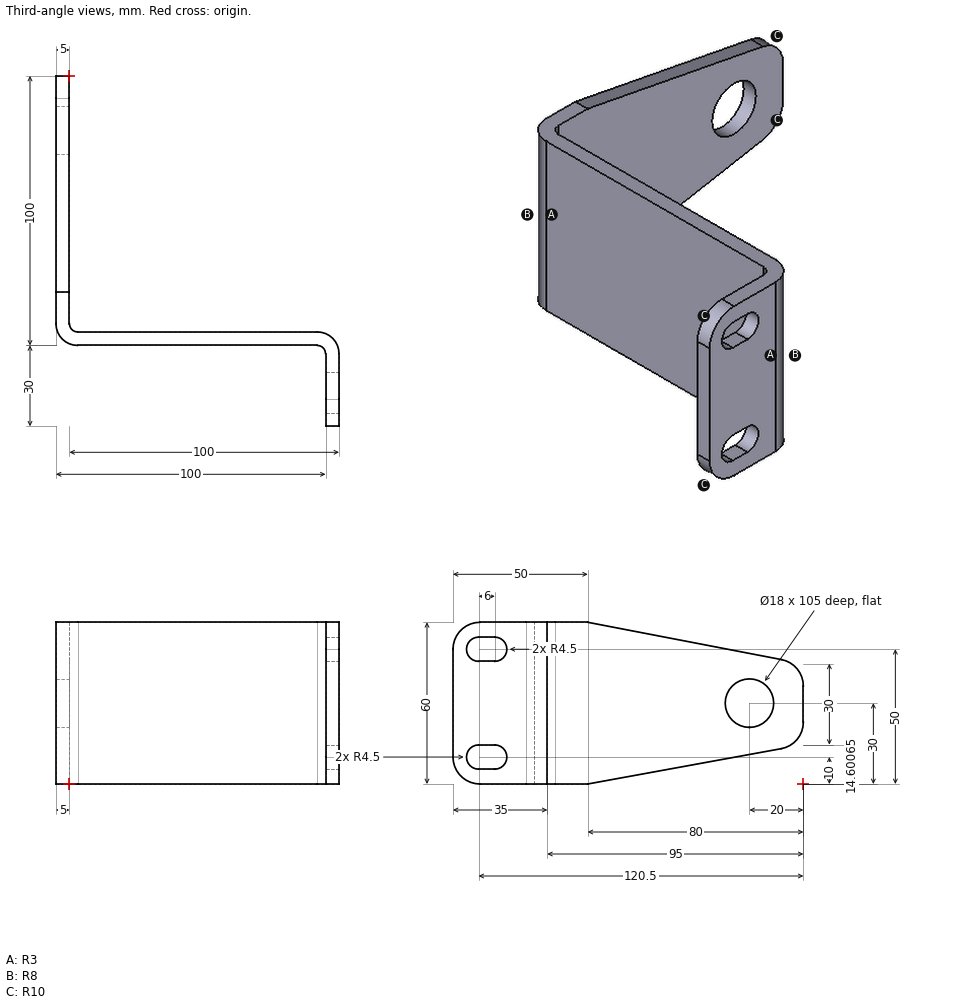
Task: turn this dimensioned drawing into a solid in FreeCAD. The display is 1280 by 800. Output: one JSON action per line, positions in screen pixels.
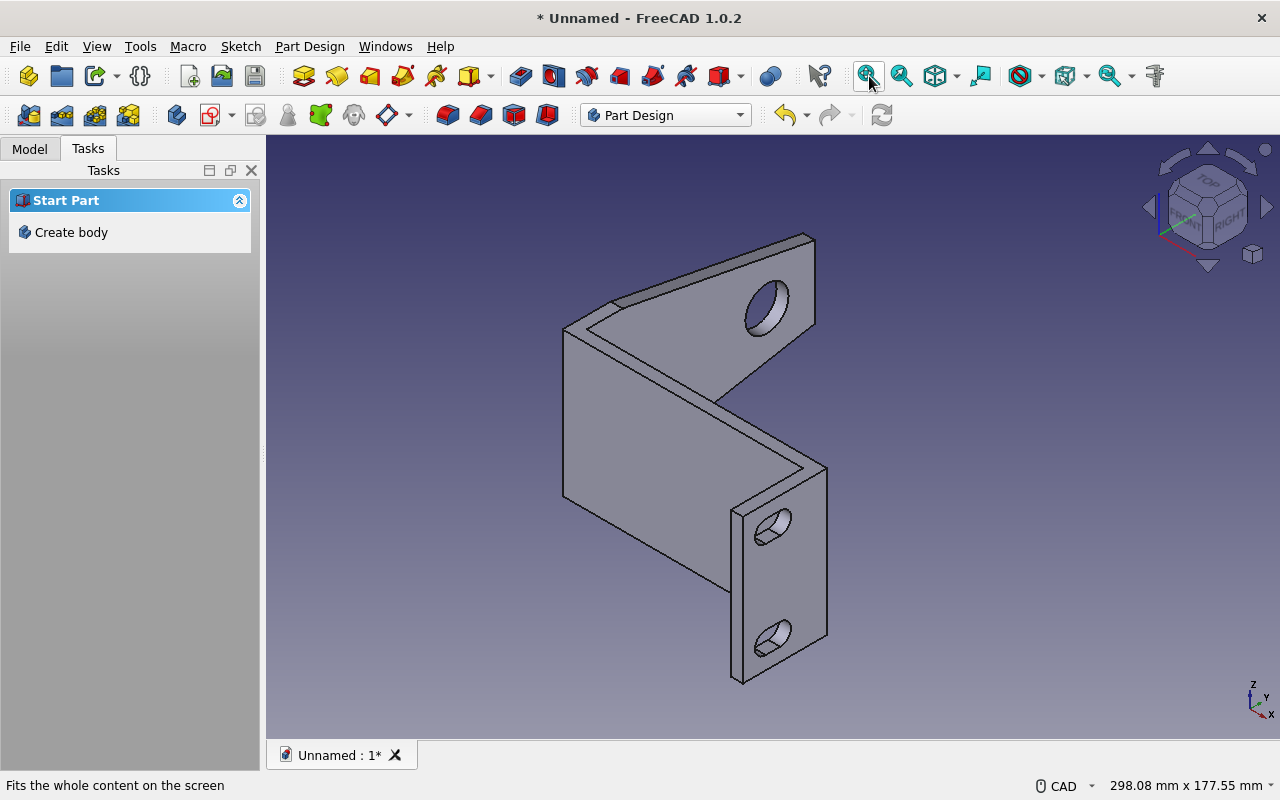
{"action": "key", "text": "2"}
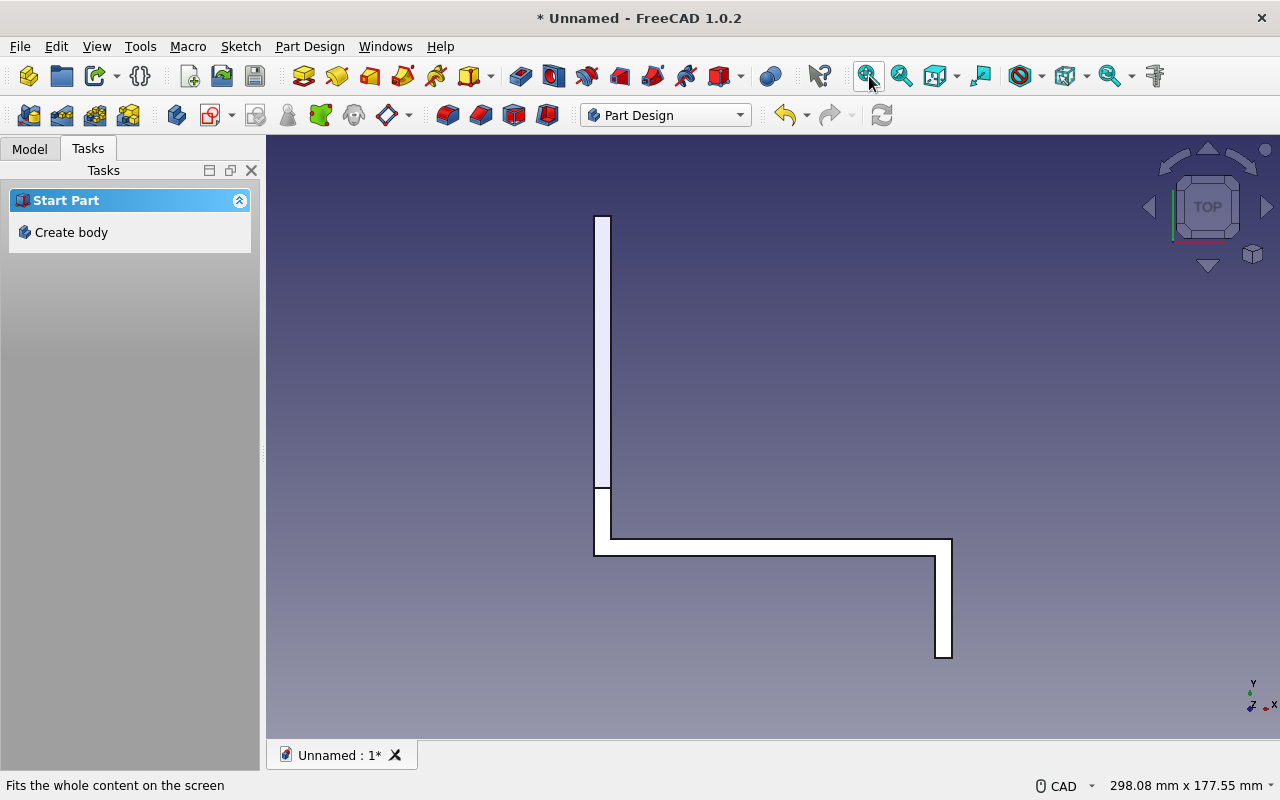
{"action": "key", "text": "1"}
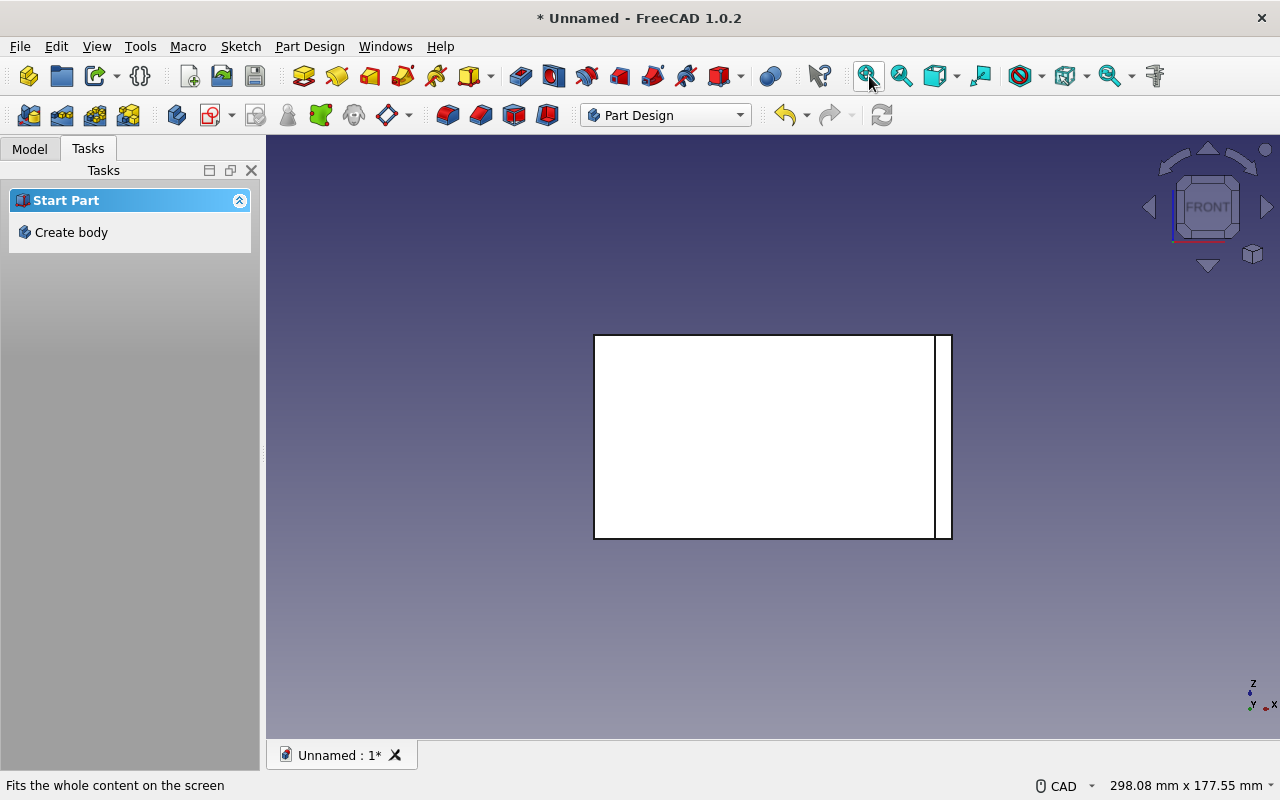
{"action": "left_click", "coordinate": [869, 76]}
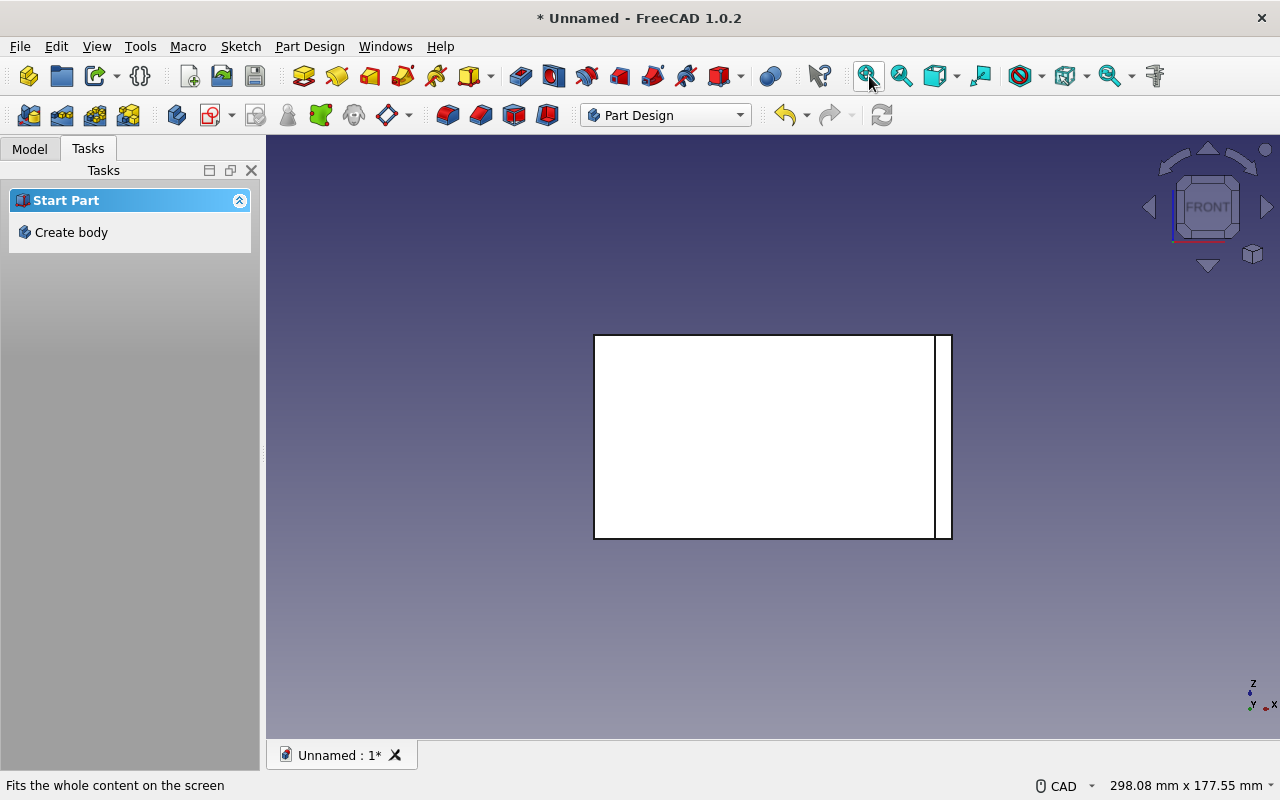
{"action": "key", "text": "3"}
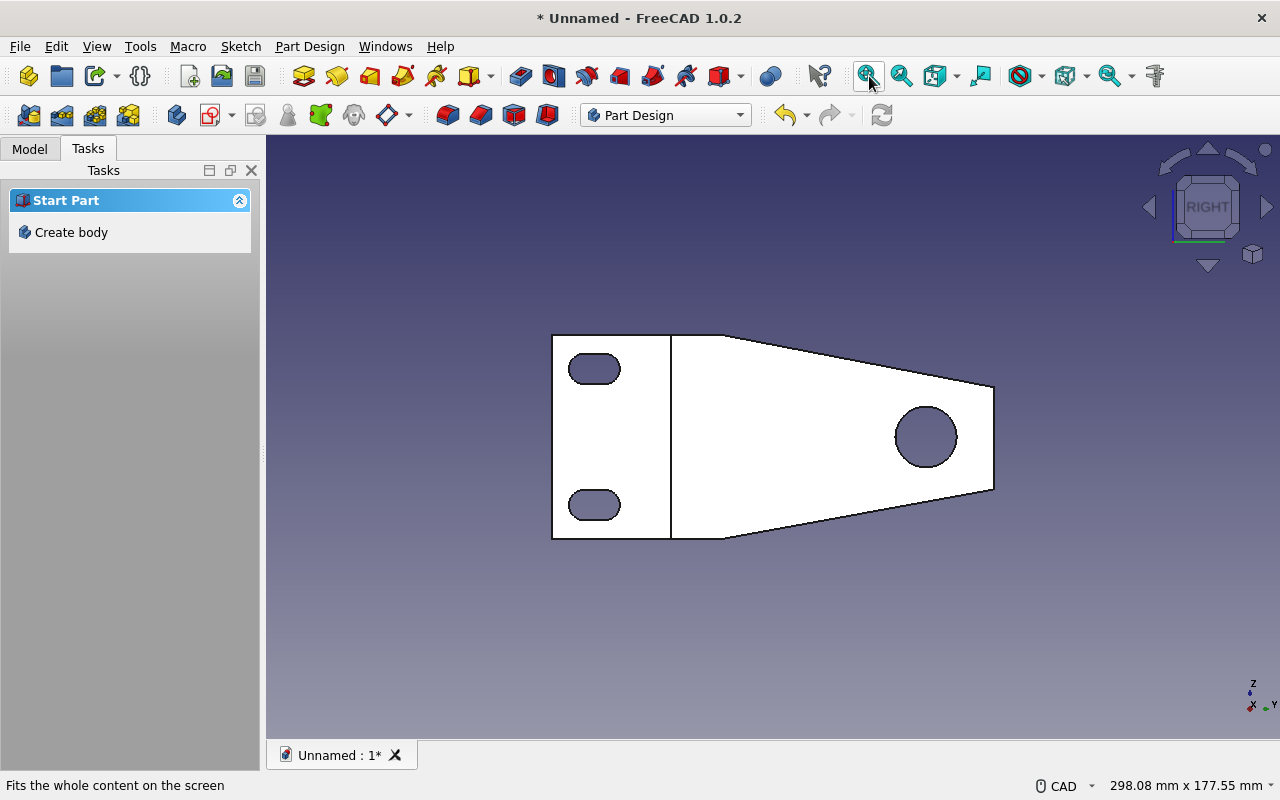
{"action": "left_click", "coordinate": [869, 76]}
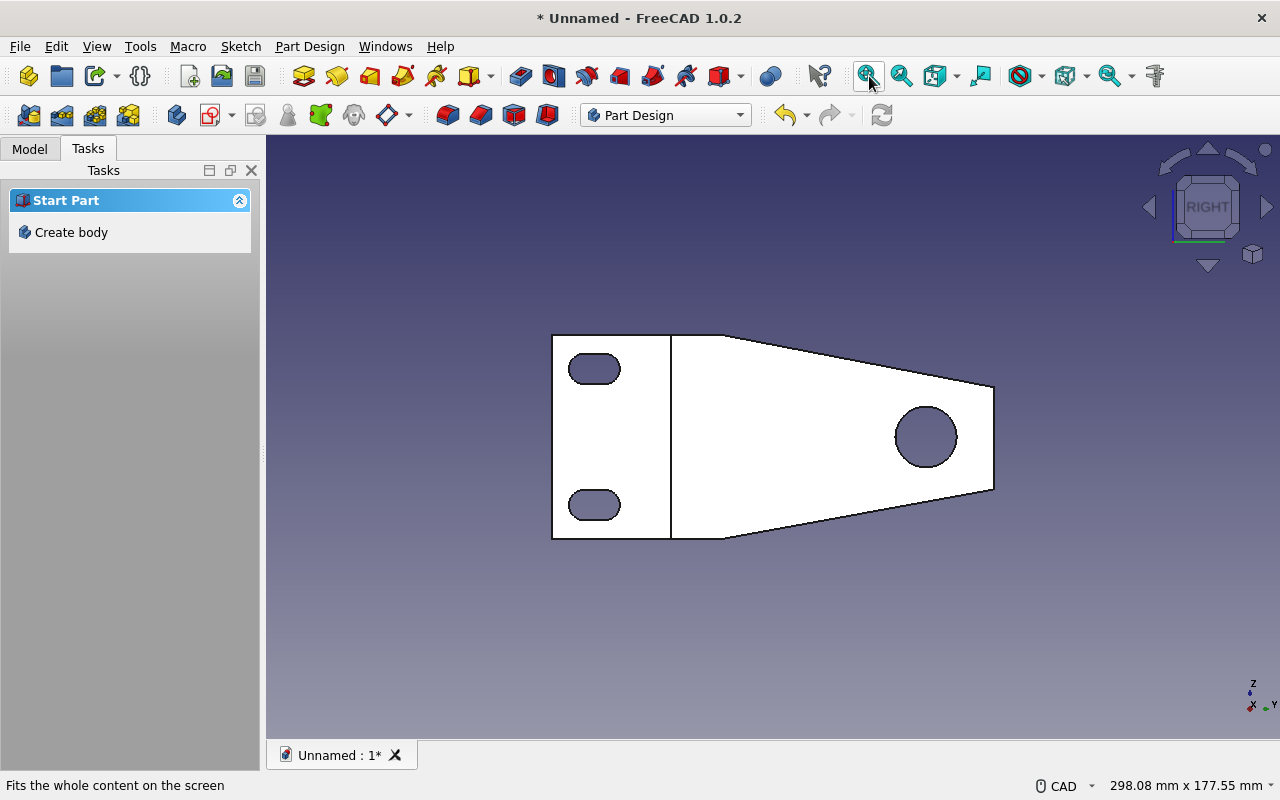
{"action": "key", "text": "5"}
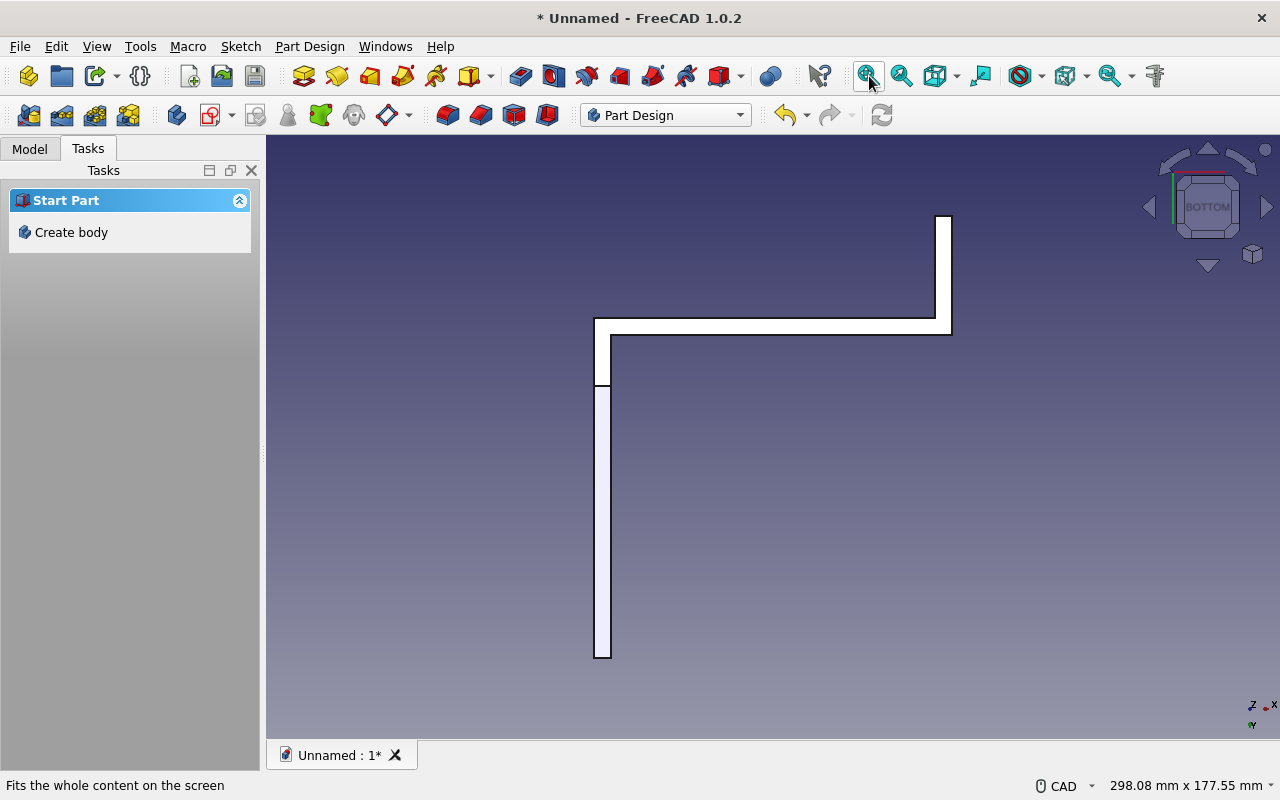
{"action": "key", "text": "4"}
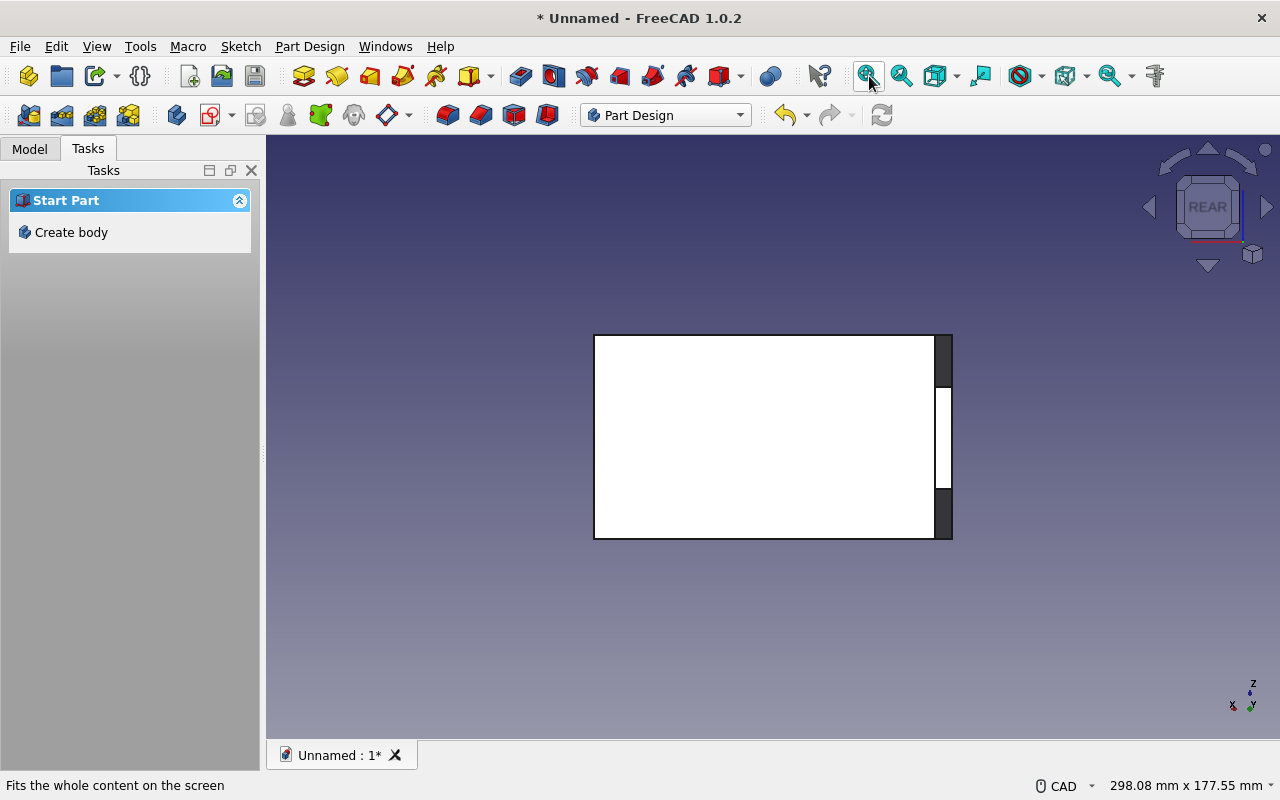
{"action": "left_click", "coordinate": [869, 76]}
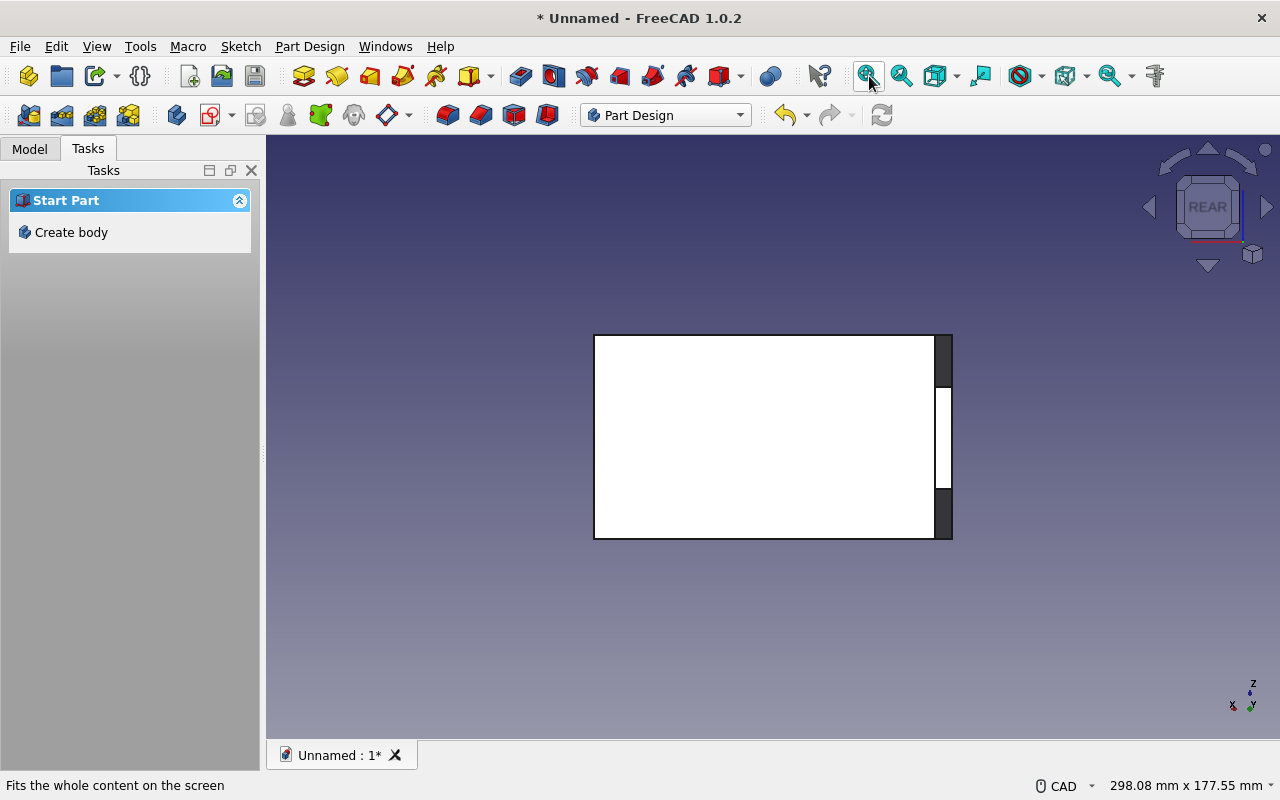
{"action": "key", "text": "6"}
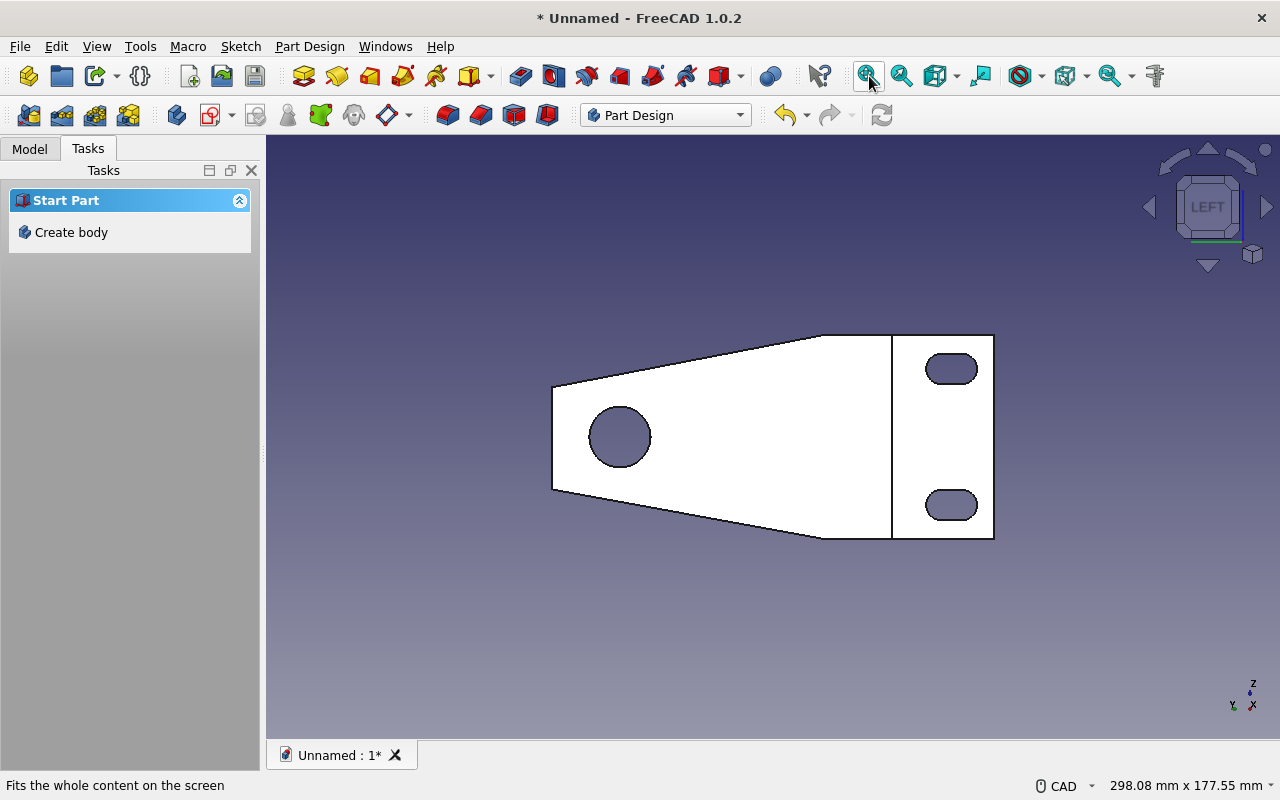
{"action": "left_click", "coordinate": [869, 76]}